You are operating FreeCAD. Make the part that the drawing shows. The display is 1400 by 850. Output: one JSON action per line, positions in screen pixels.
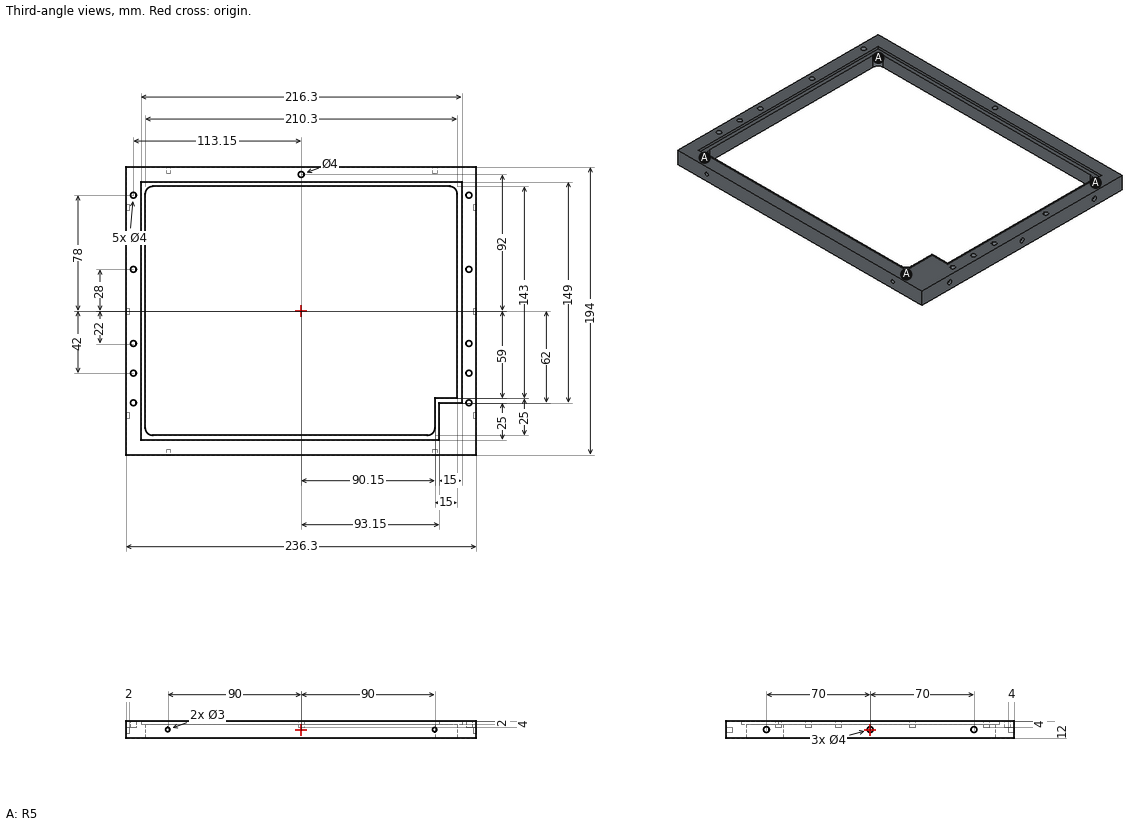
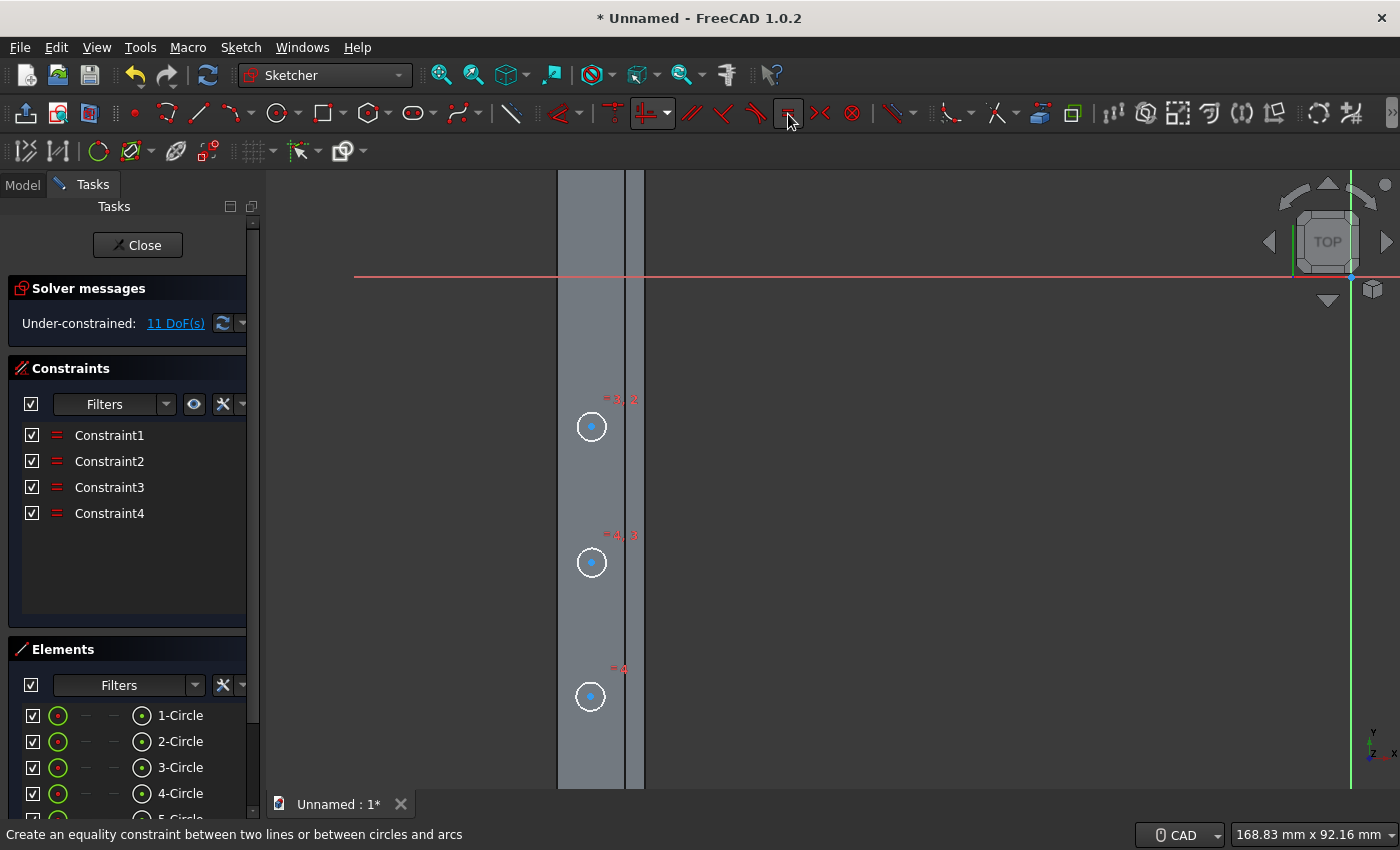
{"action": "left_click", "coordinate": [558, 114]}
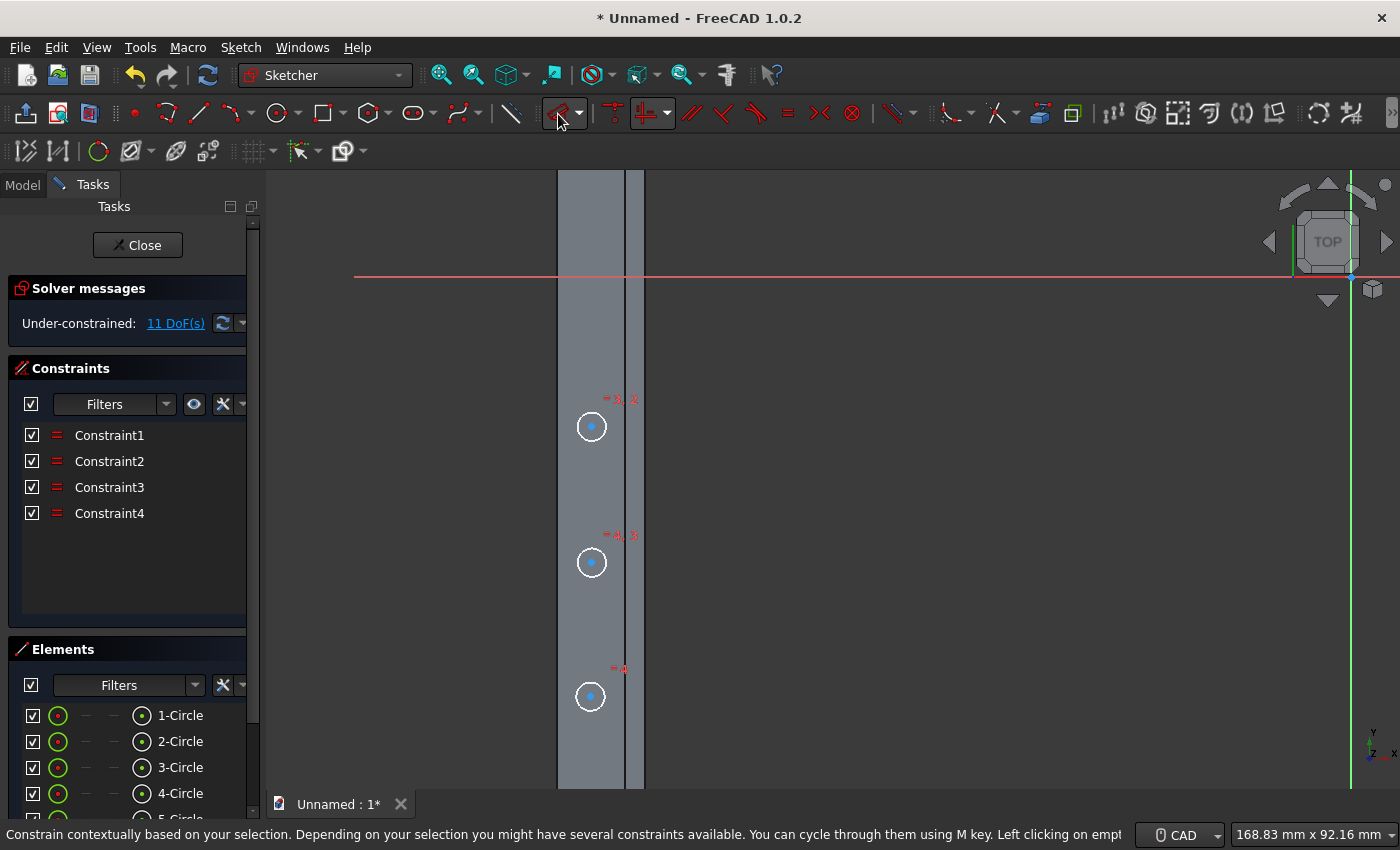
{"action": "scroll", "coordinate": [601, 688], "scroll_direction": "down", "scroll_amount": 4}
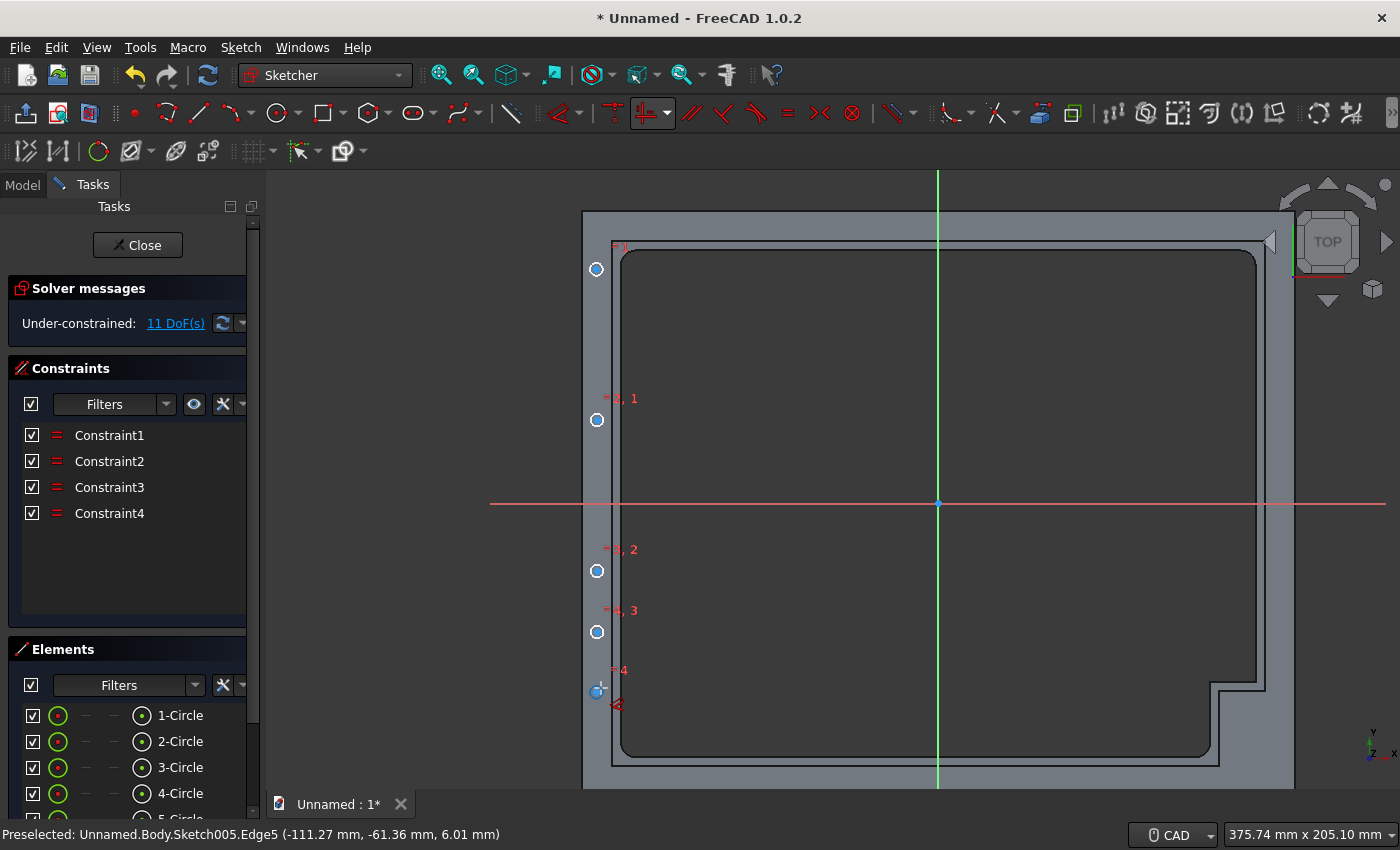
{"action": "scroll", "coordinate": [601, 265], "scroll_direction": "up", "scroll_amount": 6}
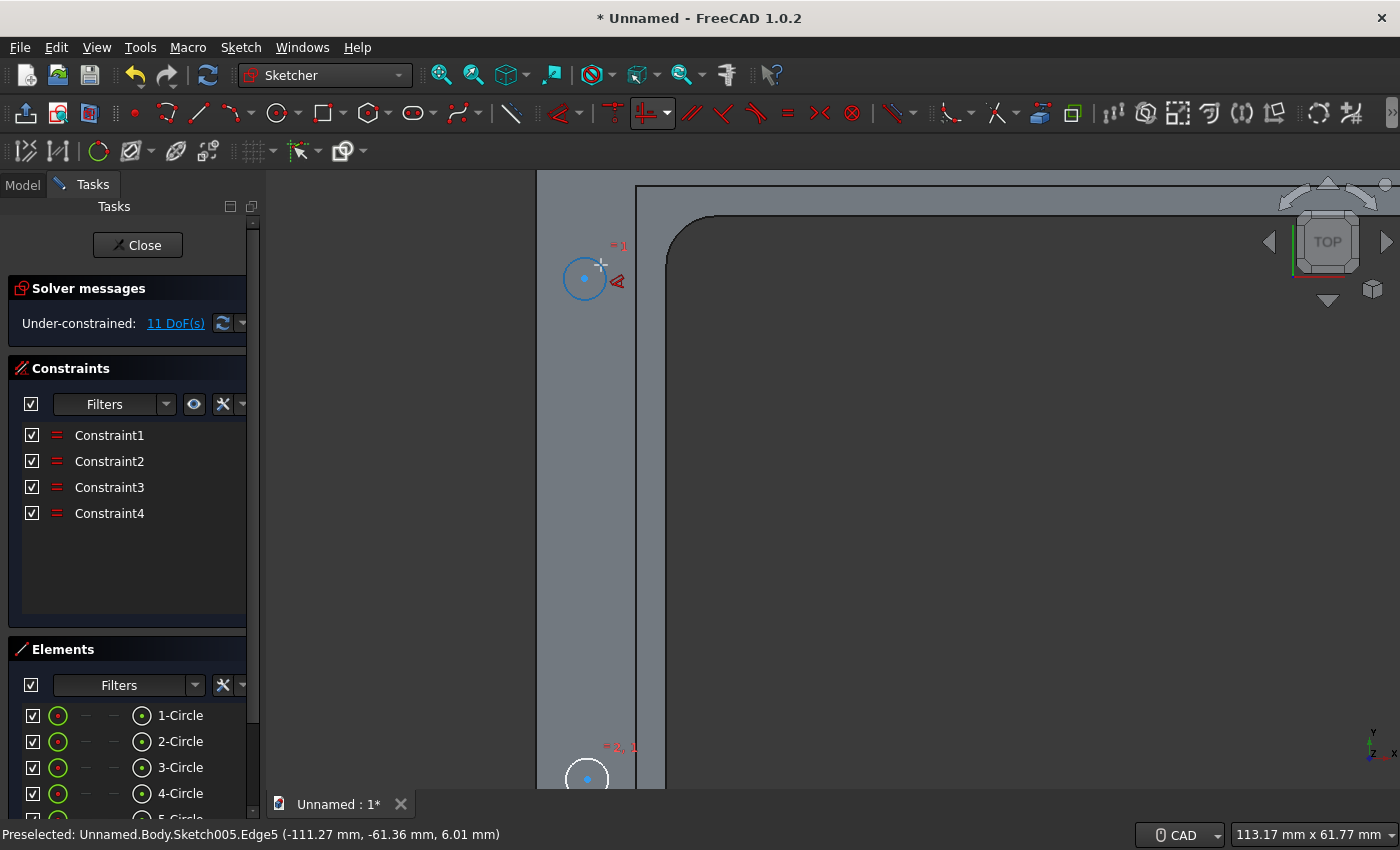
{"action": "left_click", "coordinate": [600, 264]}
{"action": "left_click", "coordinate": [623, 242]}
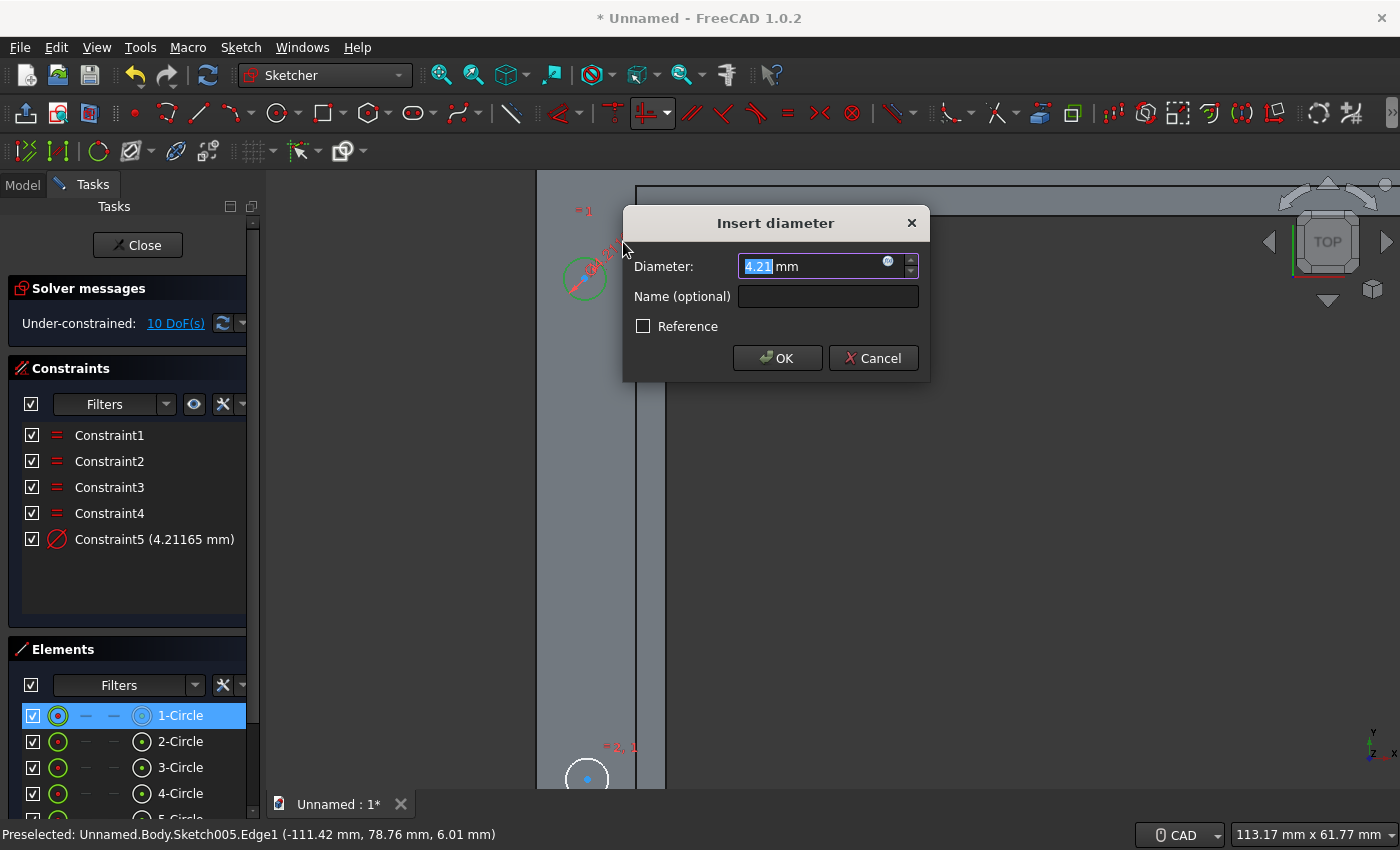
{"action": "type", "text": "4"}
{"action": "key", "text": "Return"}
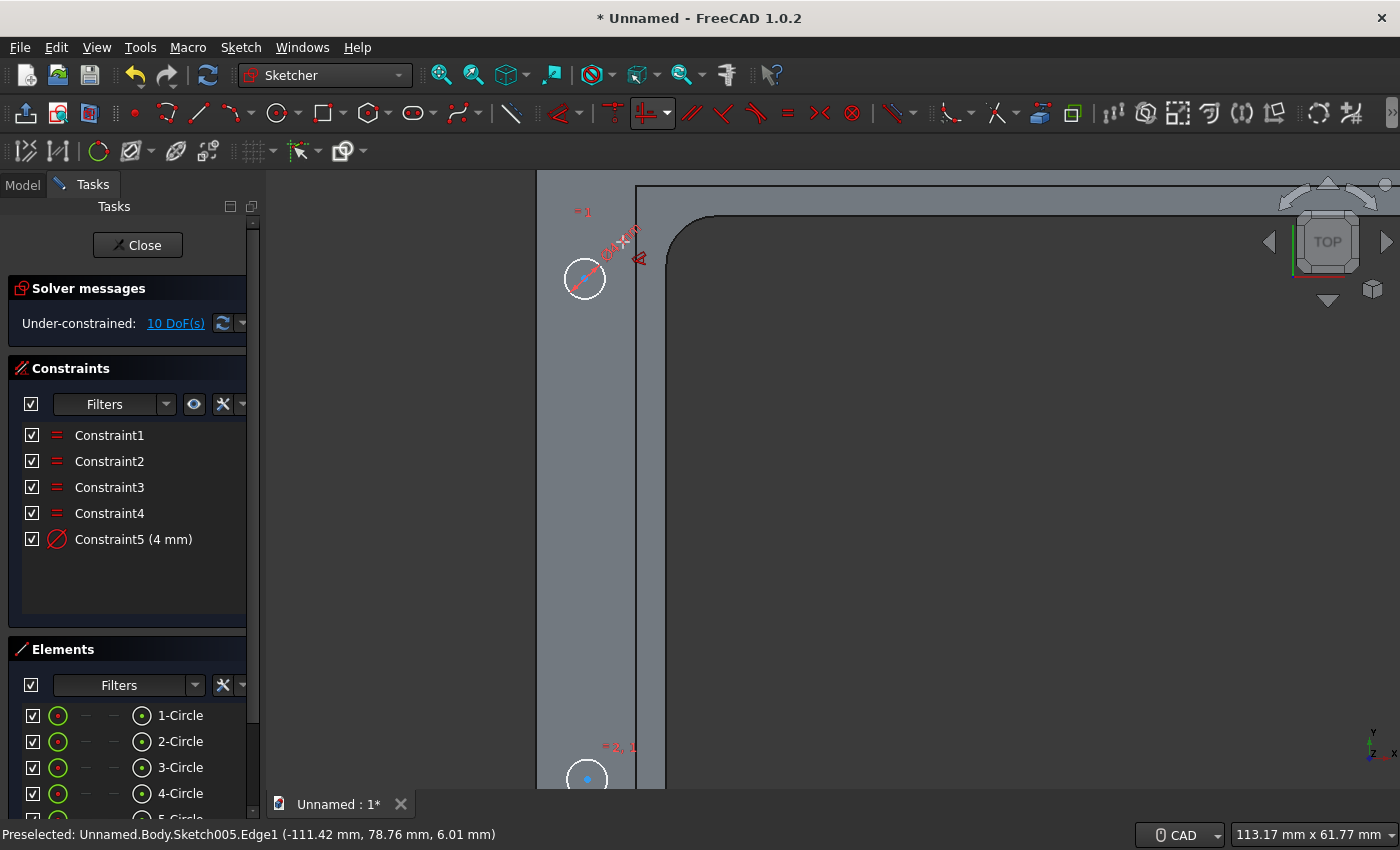
{"action": "left_click", "coordinate": [585, 279]}
{"action": "left_click", "coordinate": [551, 520]}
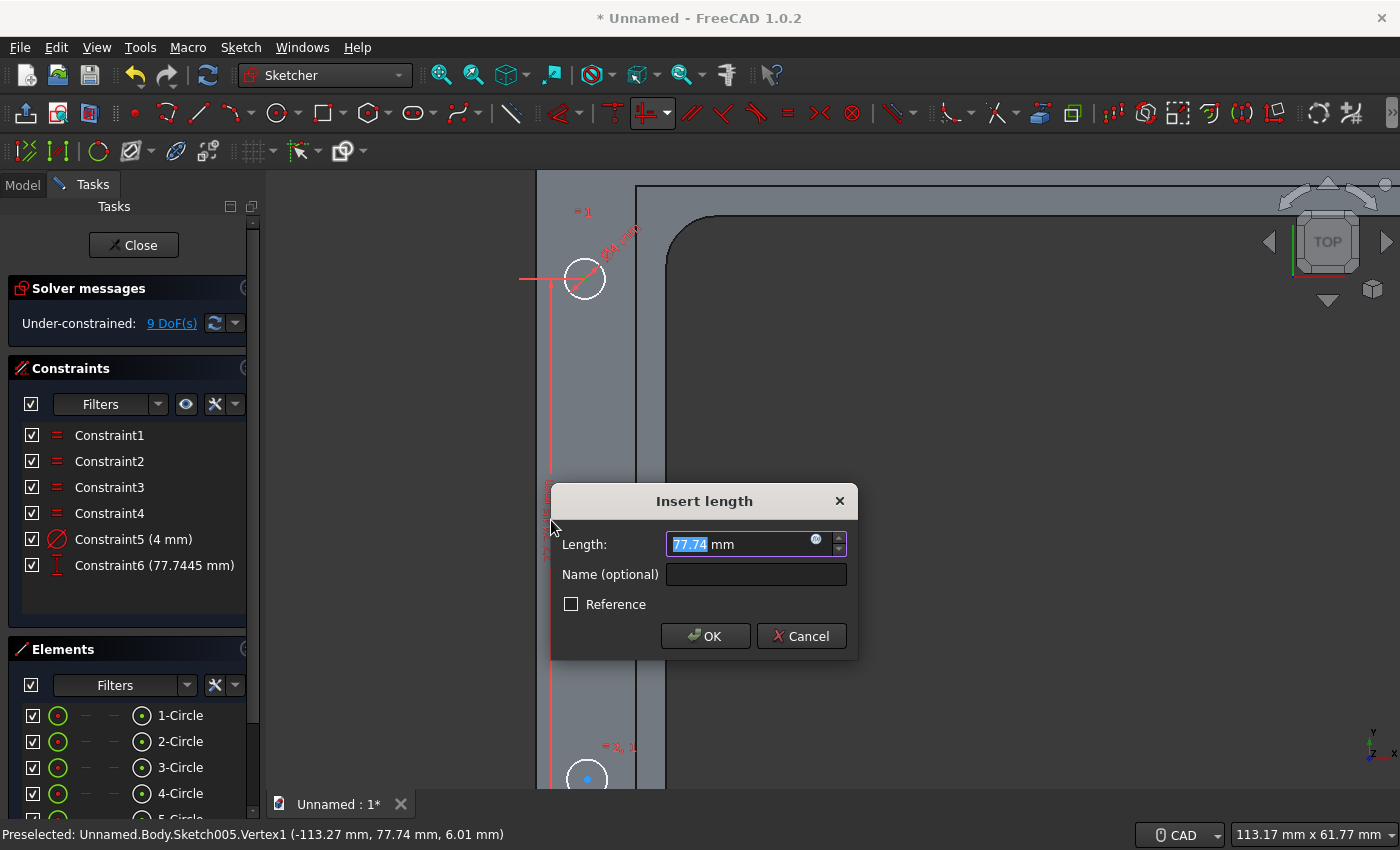
{"action": "type", "text": "78"}
{"action": "key", "text": "Return"}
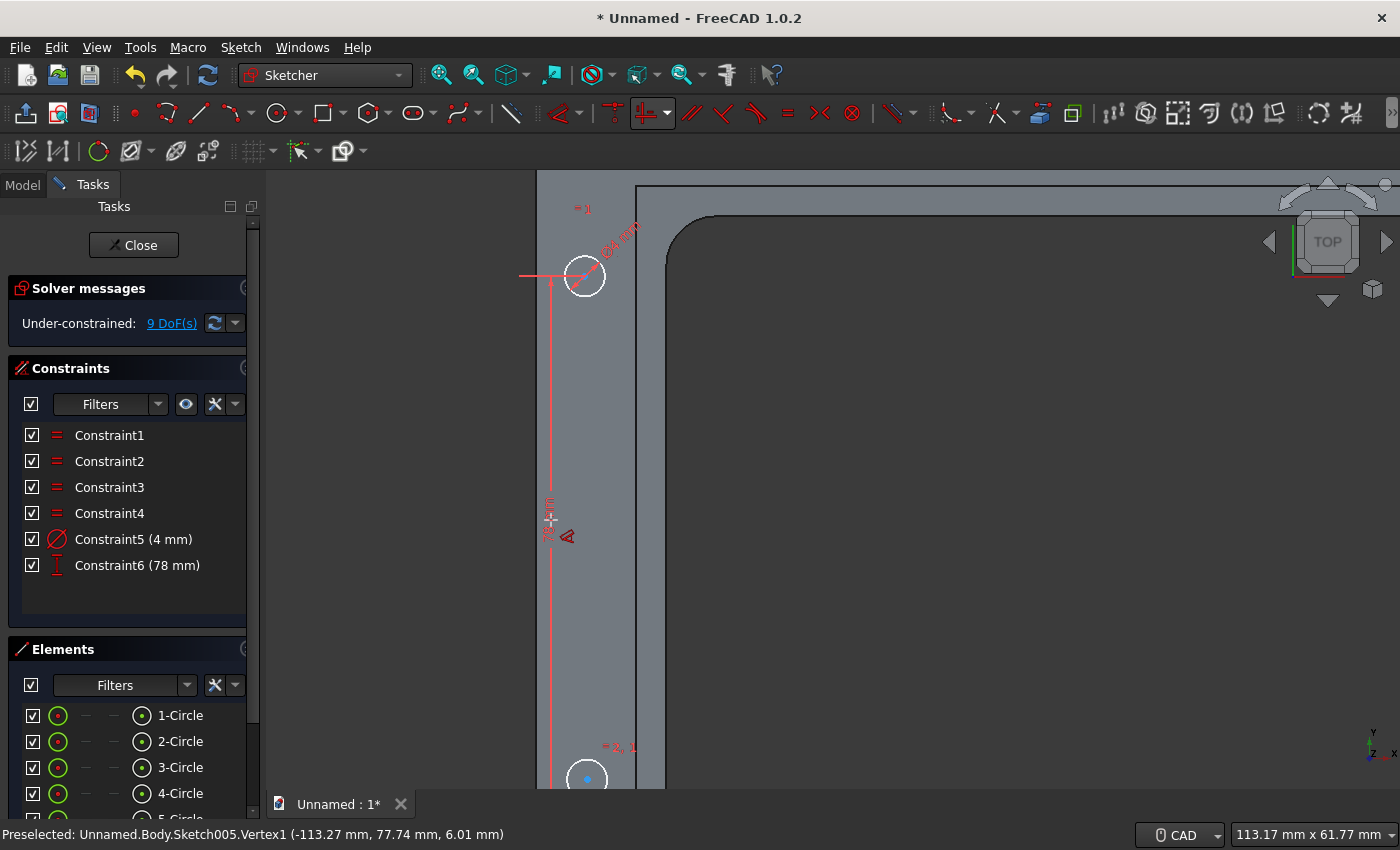
{"action": "scroll", "coordinate": [601, 265], "scroll_direction": "down", "scroll_amount": 6}